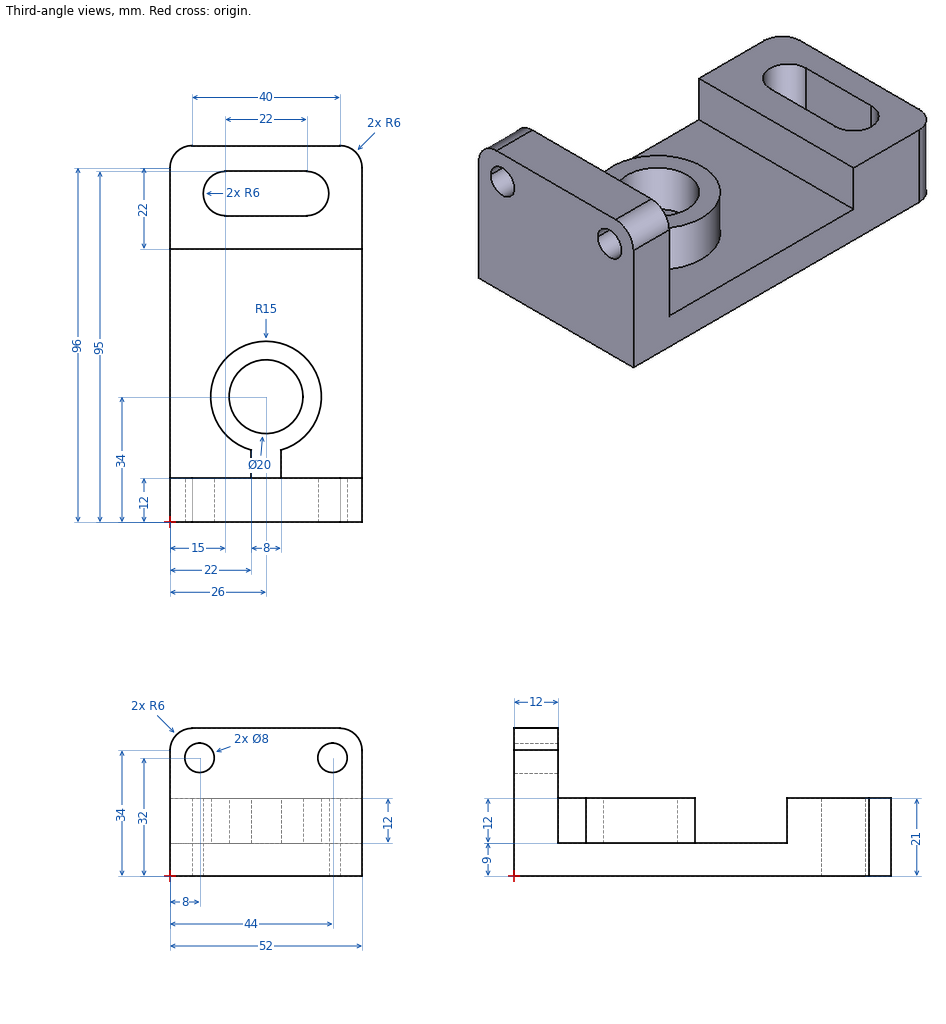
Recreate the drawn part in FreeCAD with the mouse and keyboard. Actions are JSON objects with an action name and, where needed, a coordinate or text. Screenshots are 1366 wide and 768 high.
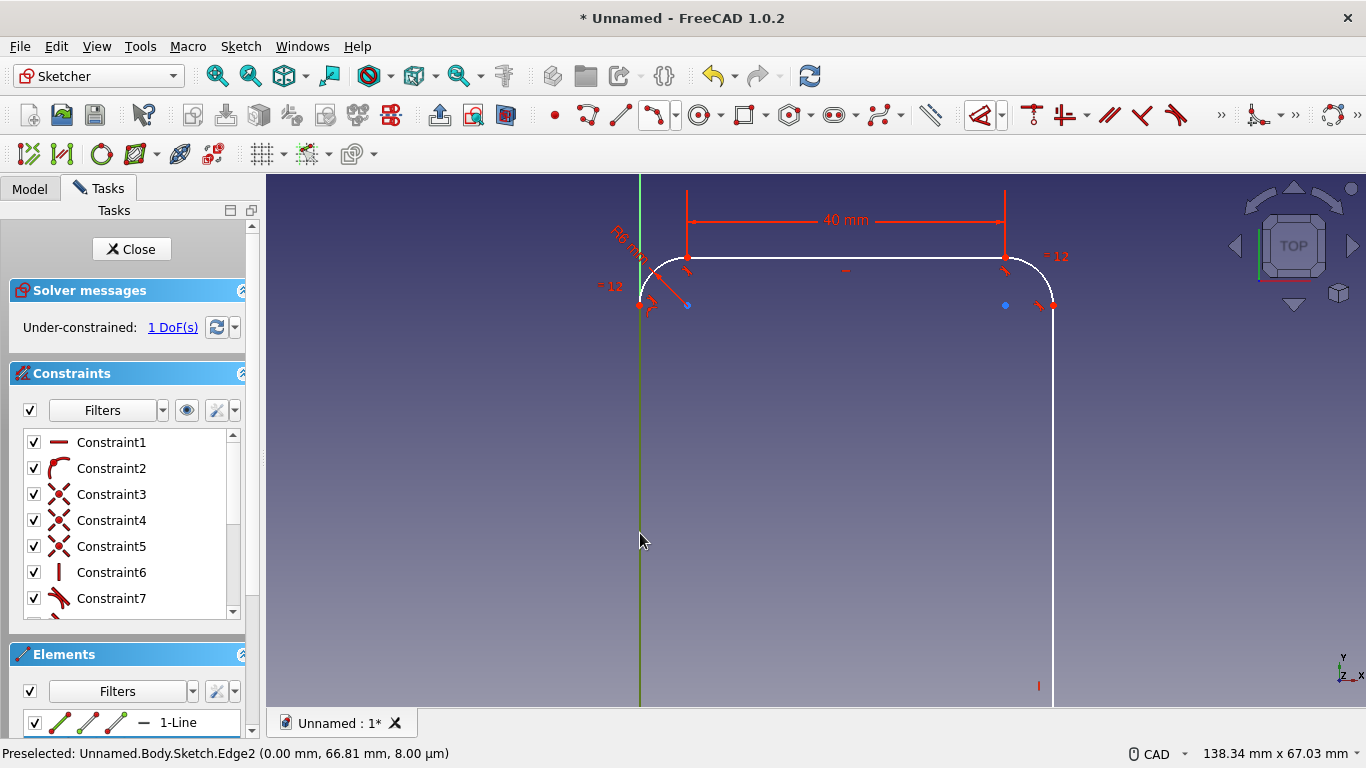
{"action": "key", "text": "i"}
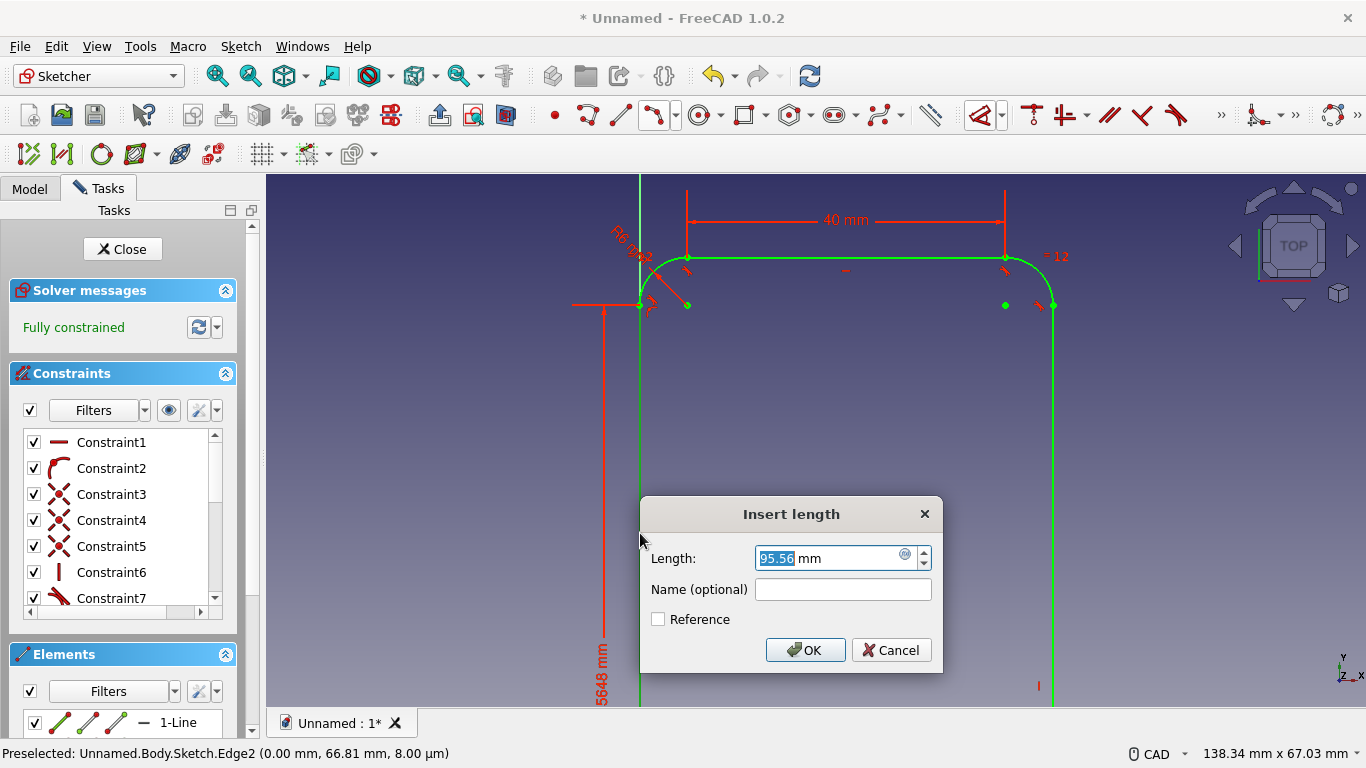
{"action": "type", "text": "96"}
{"action": "key", "text": "Return"}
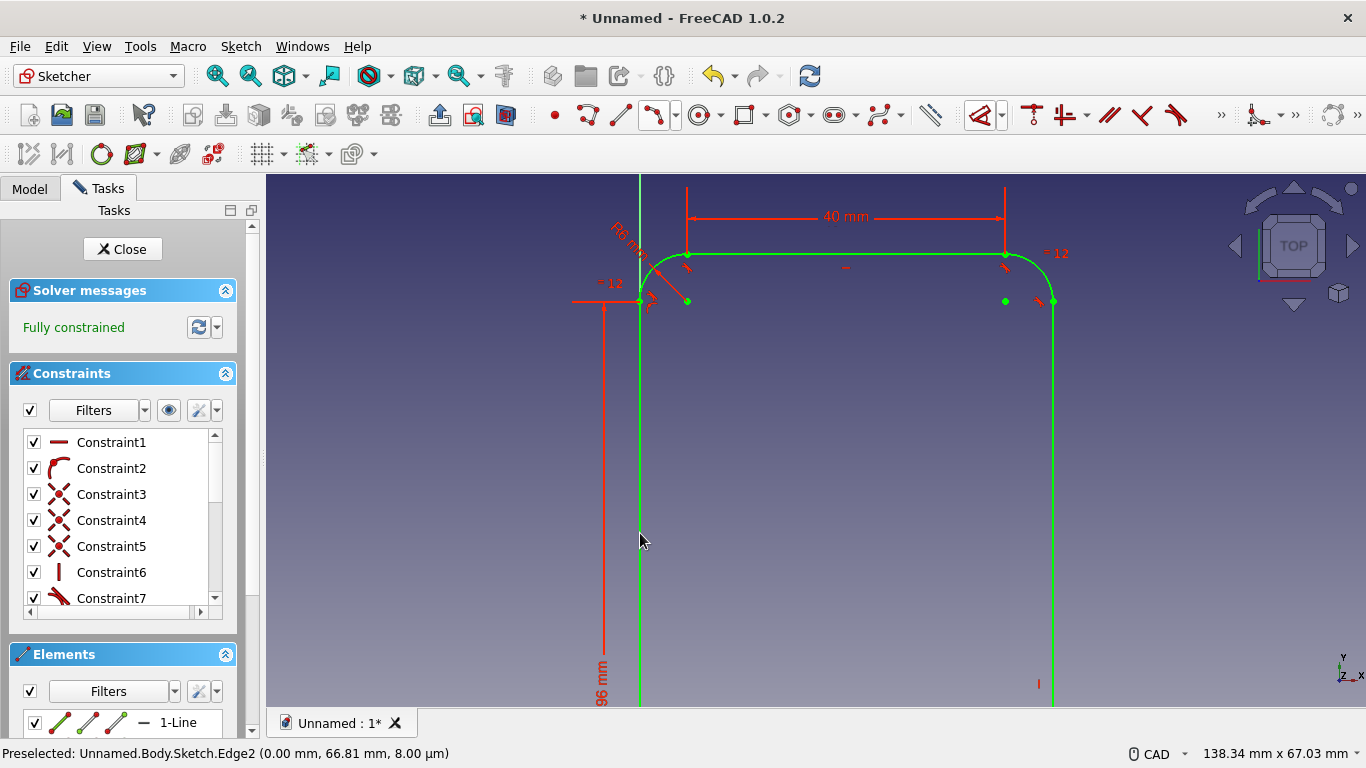
{"action": "left_click", "coordinate": [123, 249]}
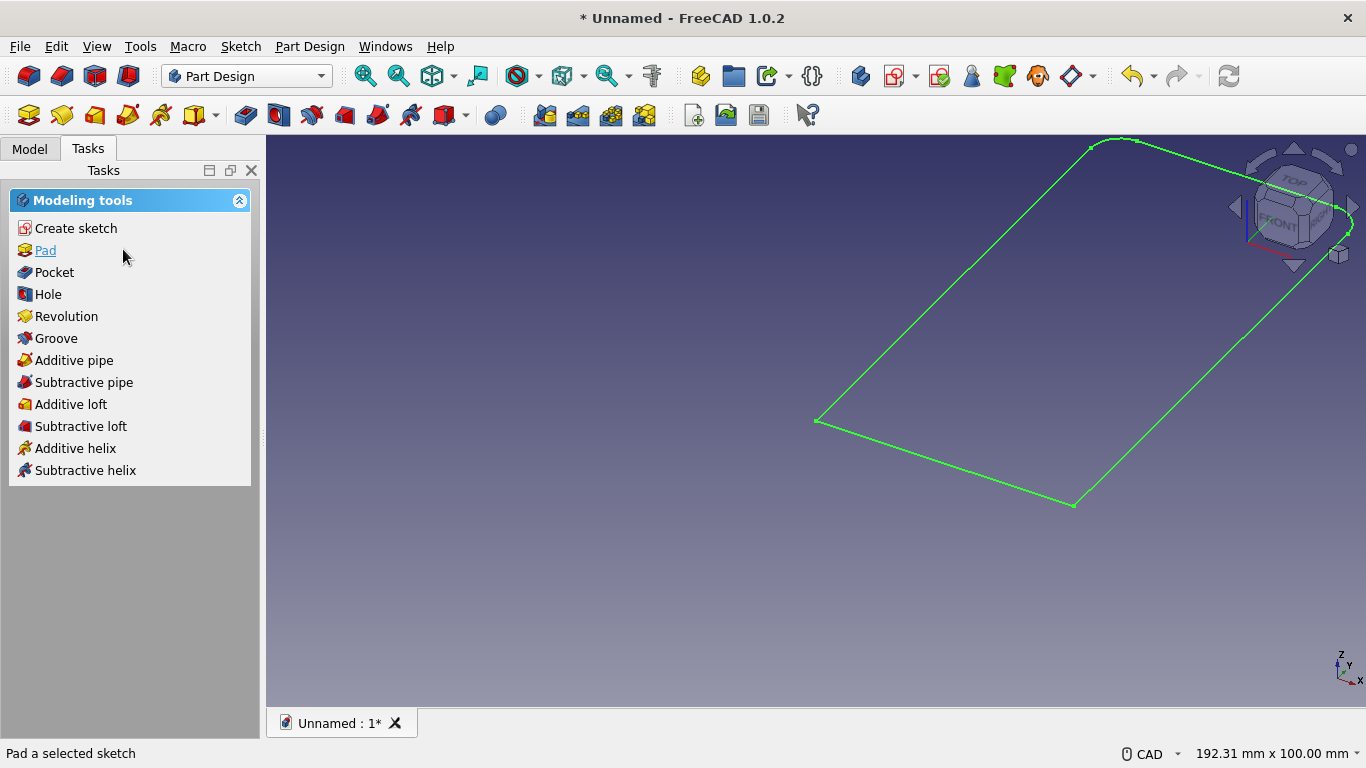
{"action": "left_click", "coordinate": [29, 116]}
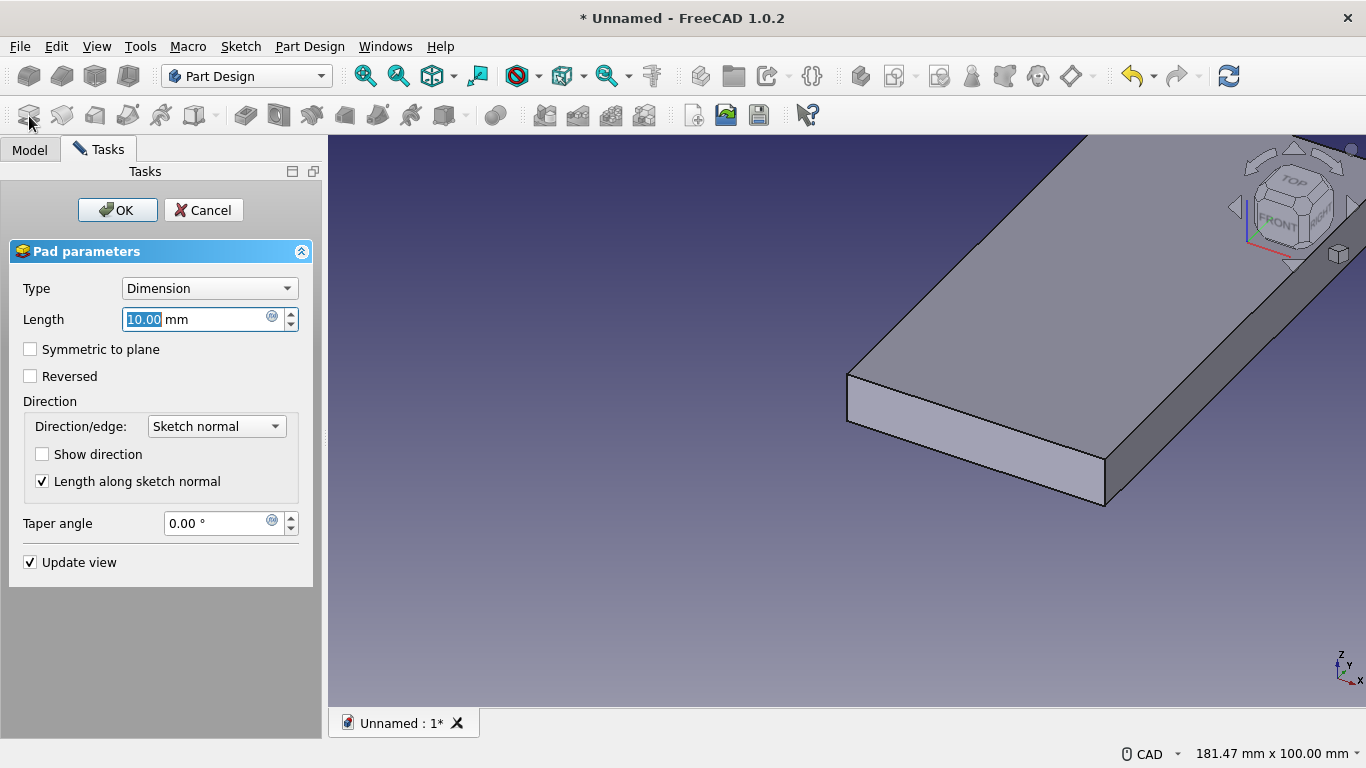
{"action": "type", "text": "9"}
{"action": "key", "text": "Tab"}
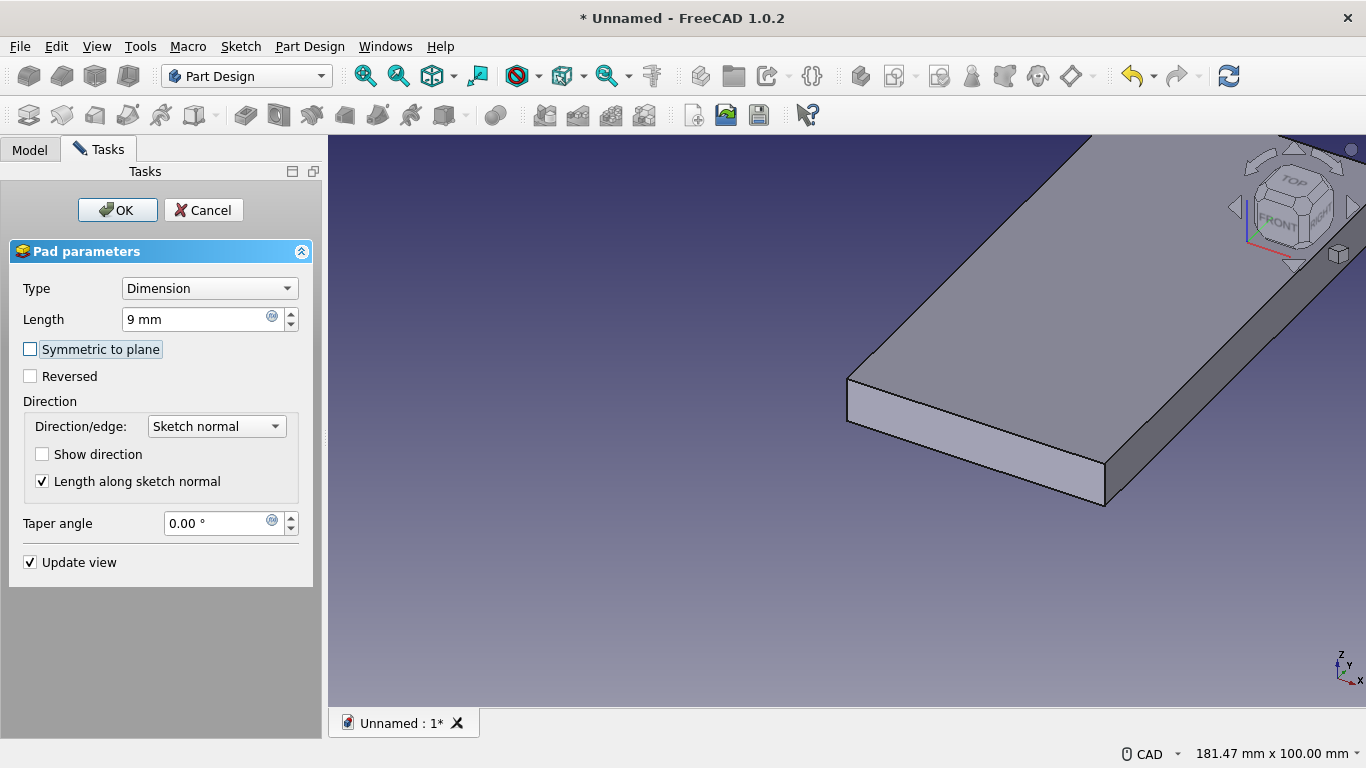
{"action": "left_click", "coordinate": [118, 210]}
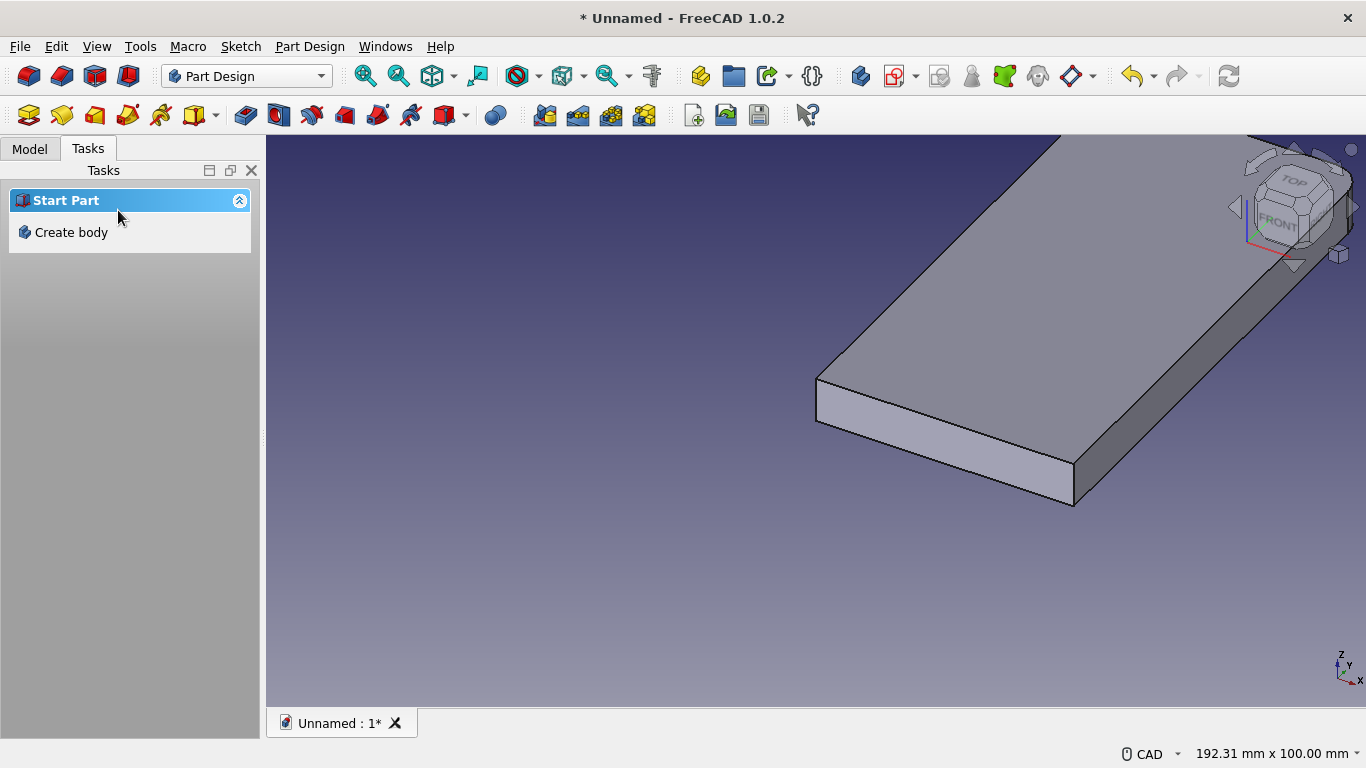
{"action": "left_click", "coordinate": [366, 76]}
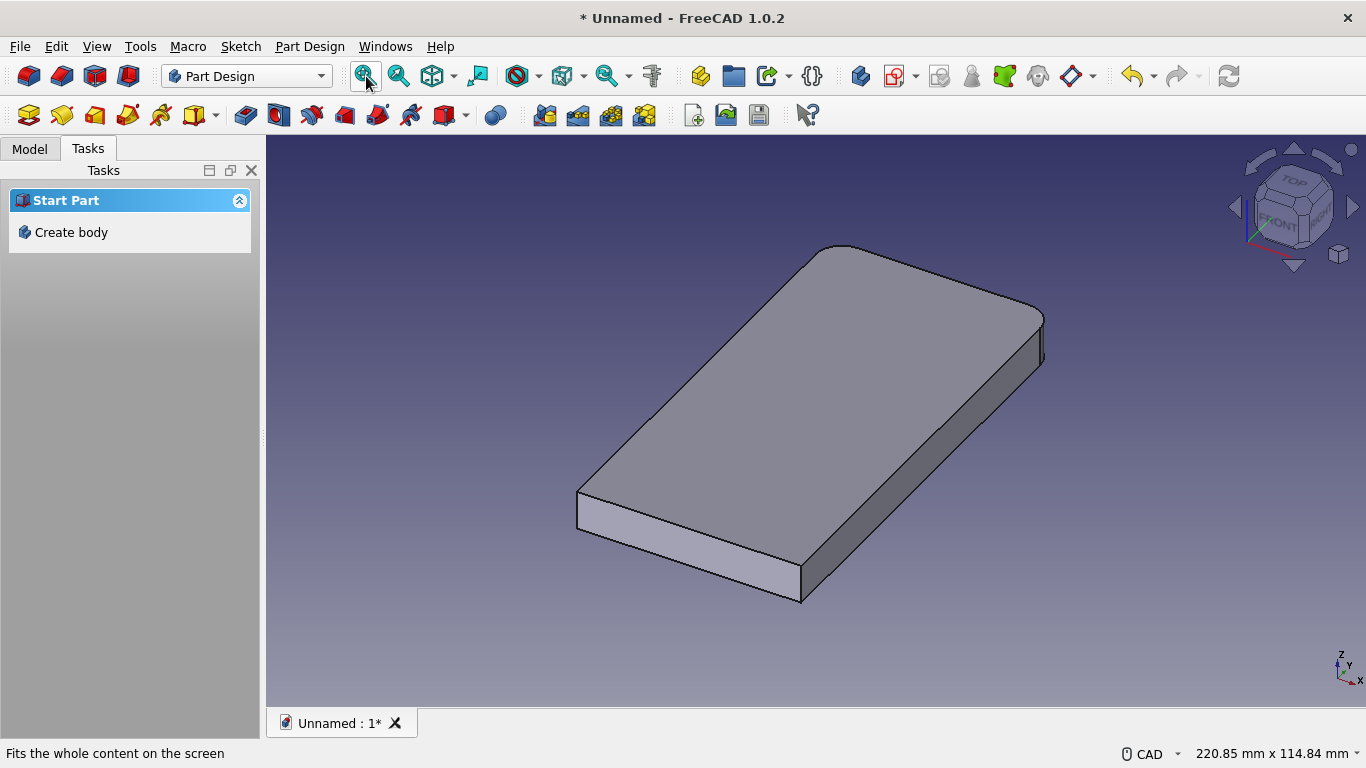
{"action": "left_click", "coordinate": [852, 366]}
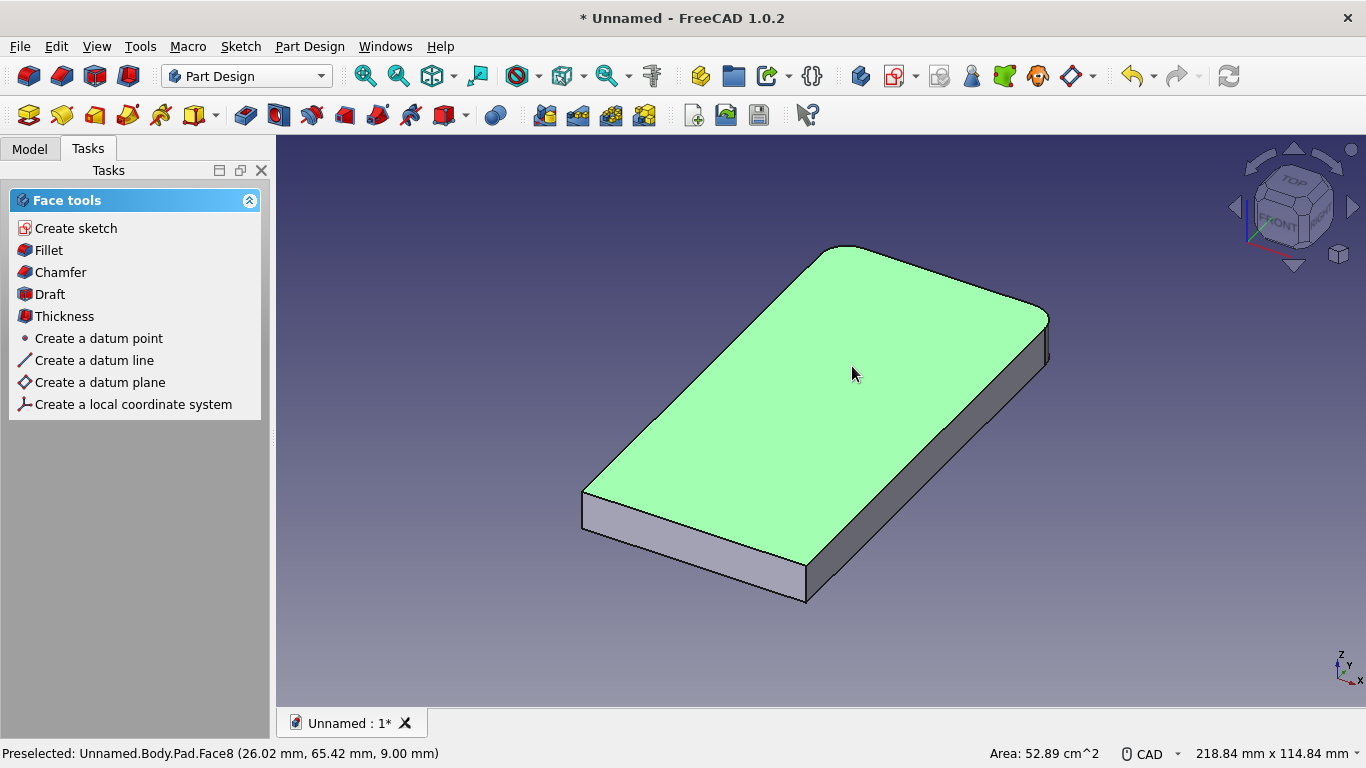
{"action": "left_click", "coordinate": [894, 76]}